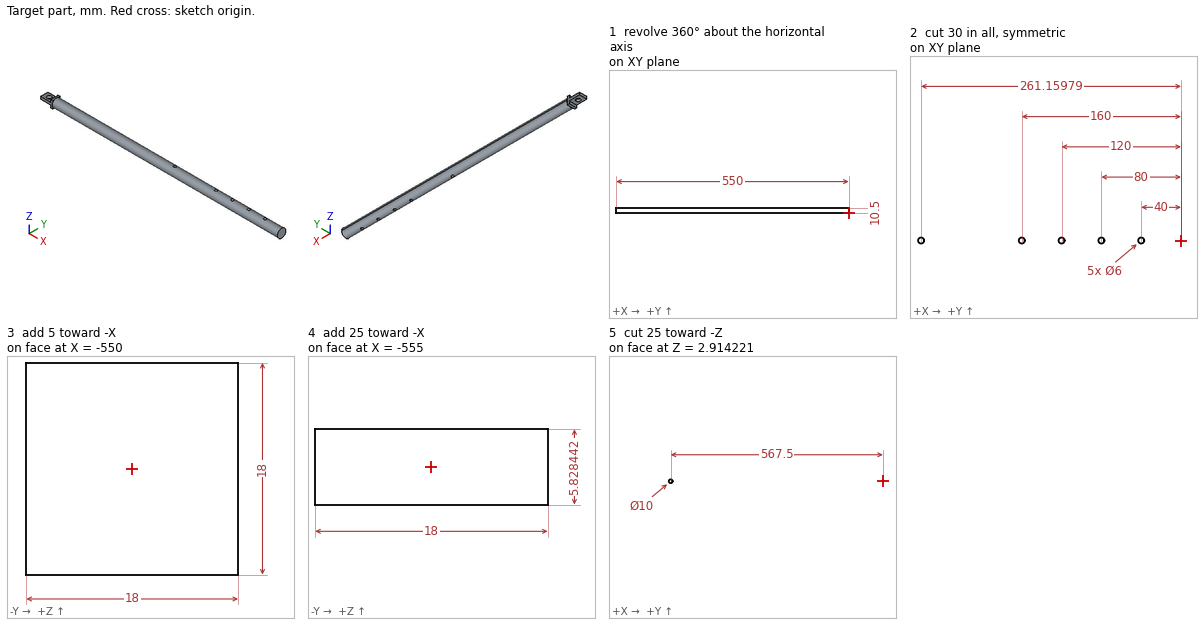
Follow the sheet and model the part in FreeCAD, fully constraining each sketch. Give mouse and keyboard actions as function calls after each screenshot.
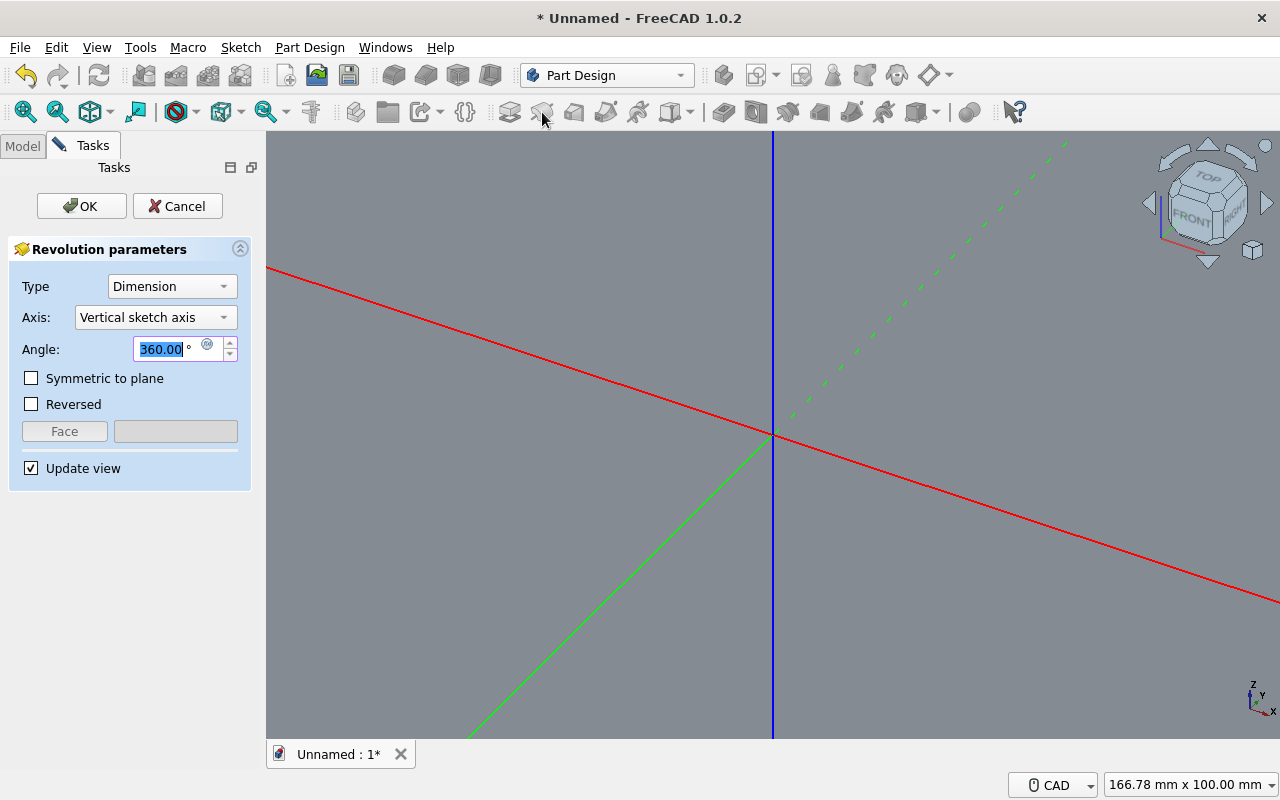
click(156, 318)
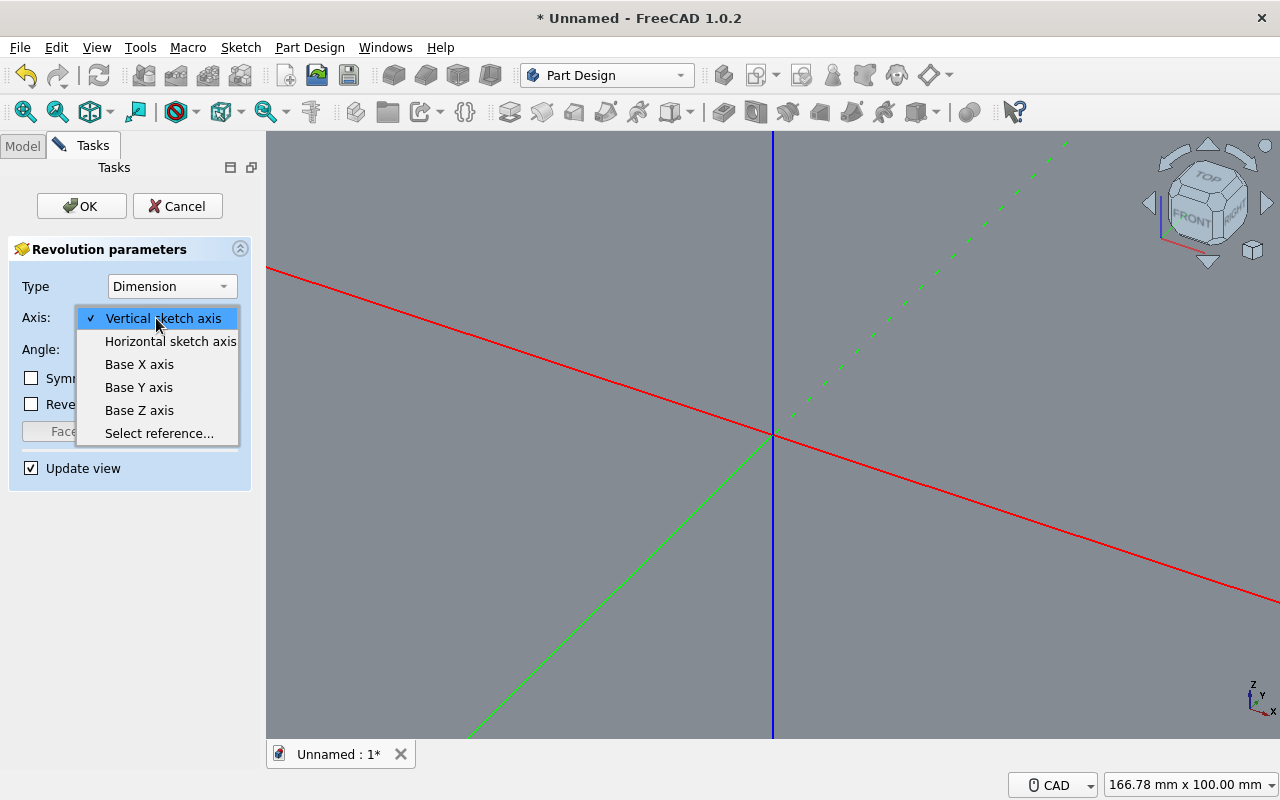
click(156, 342)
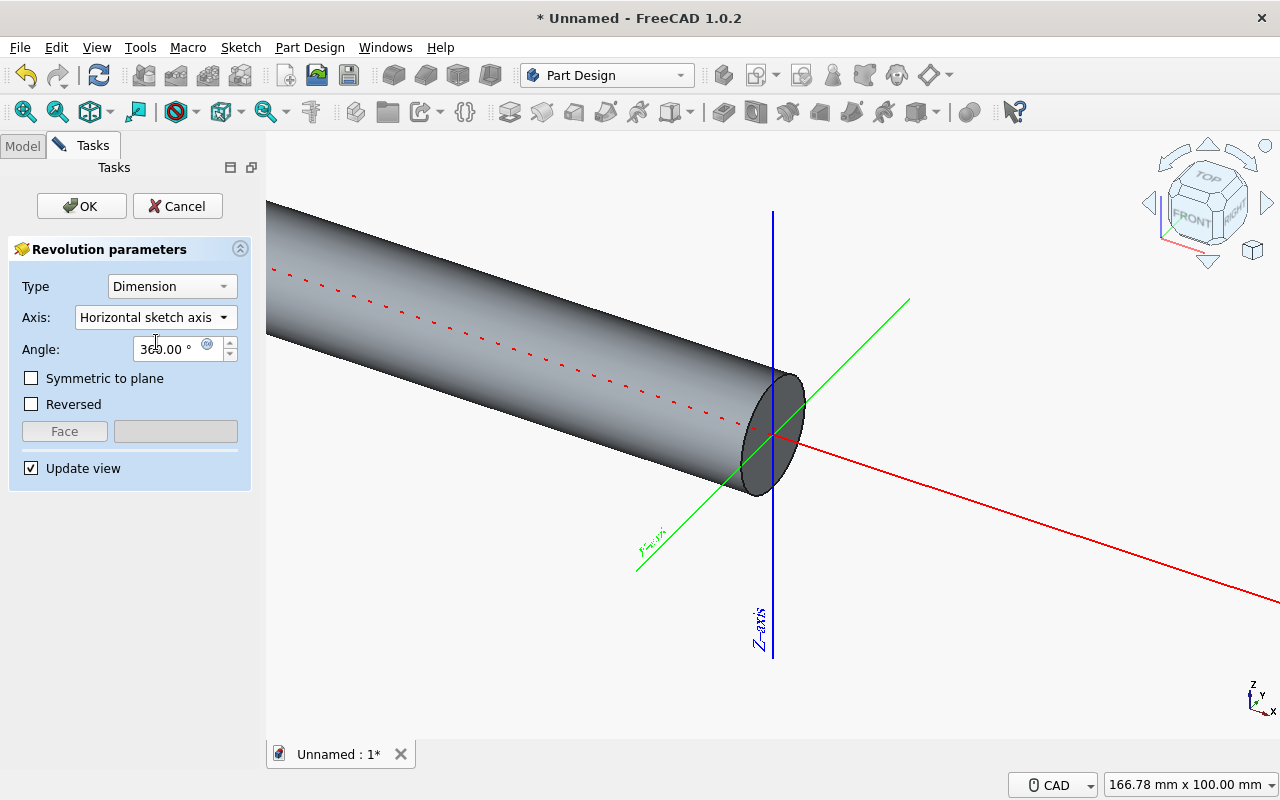
click(82, 206)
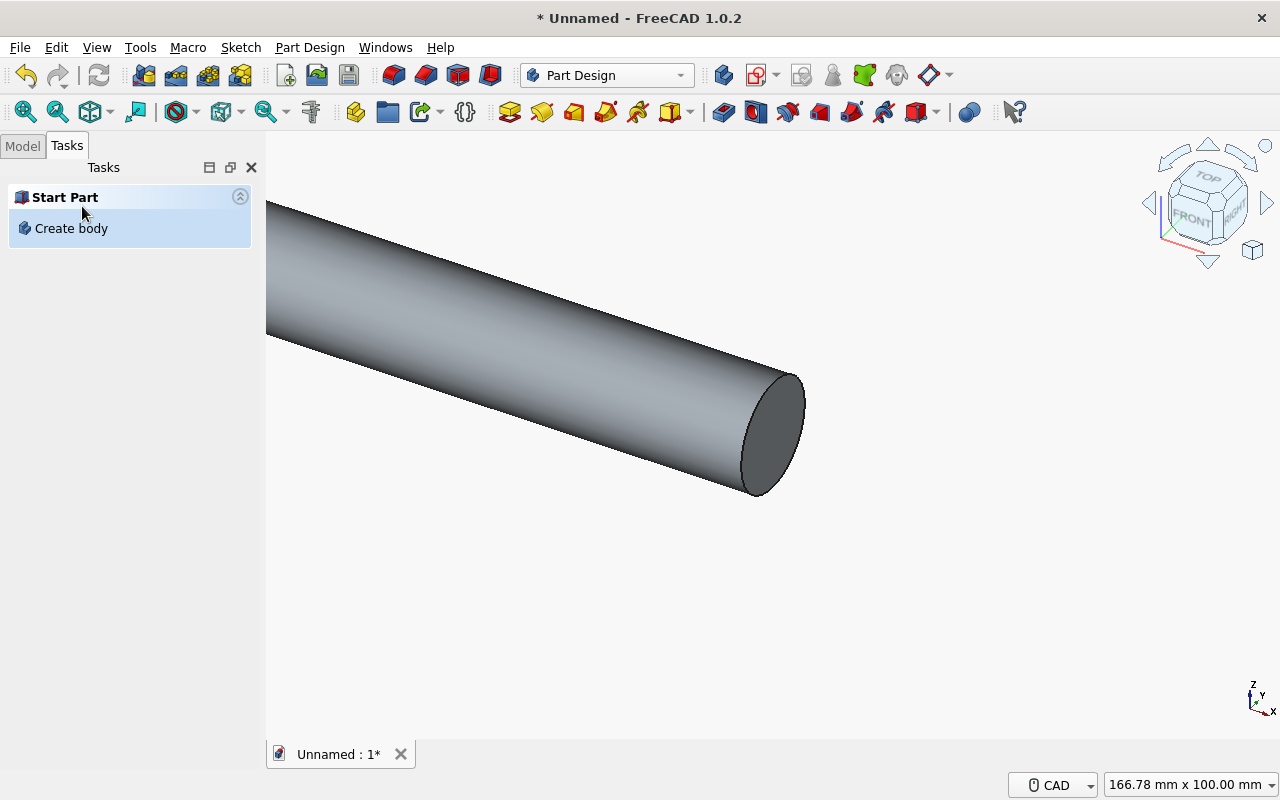
key(v)
key(f)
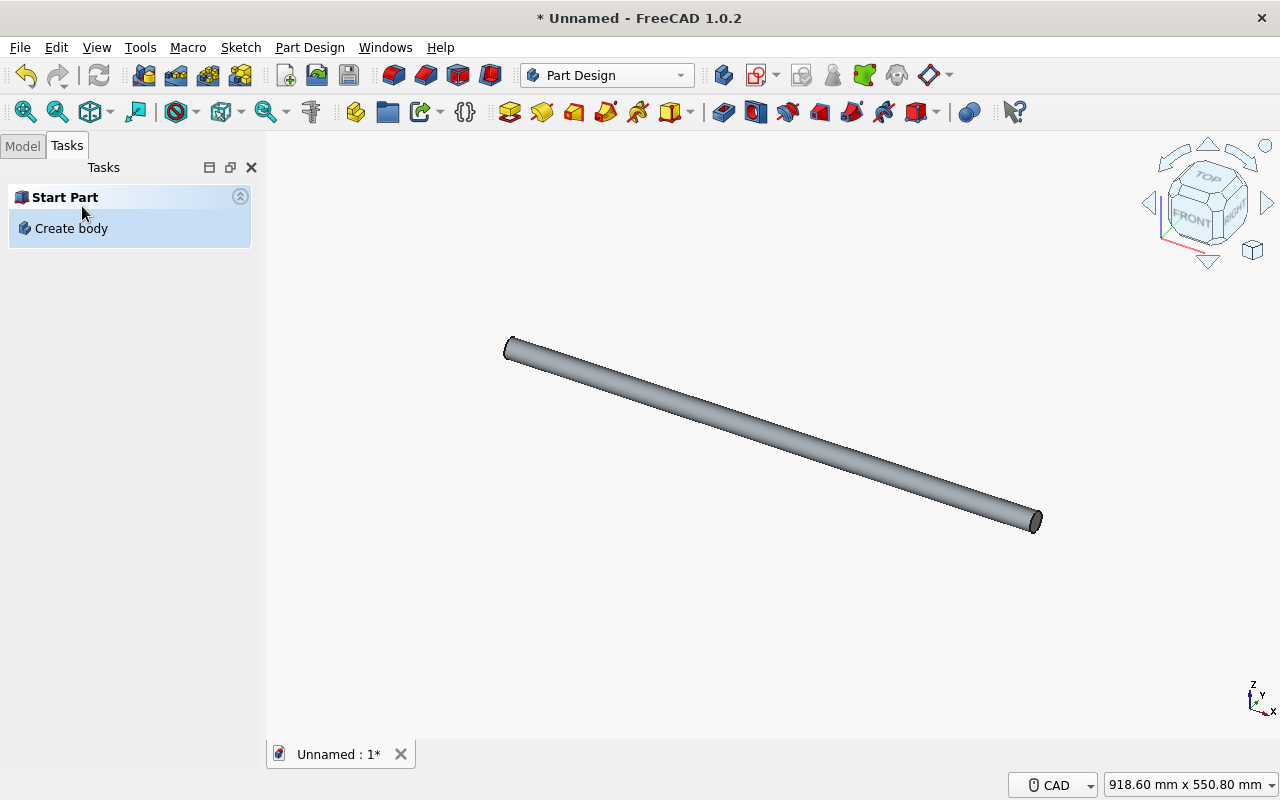
click(756, 76)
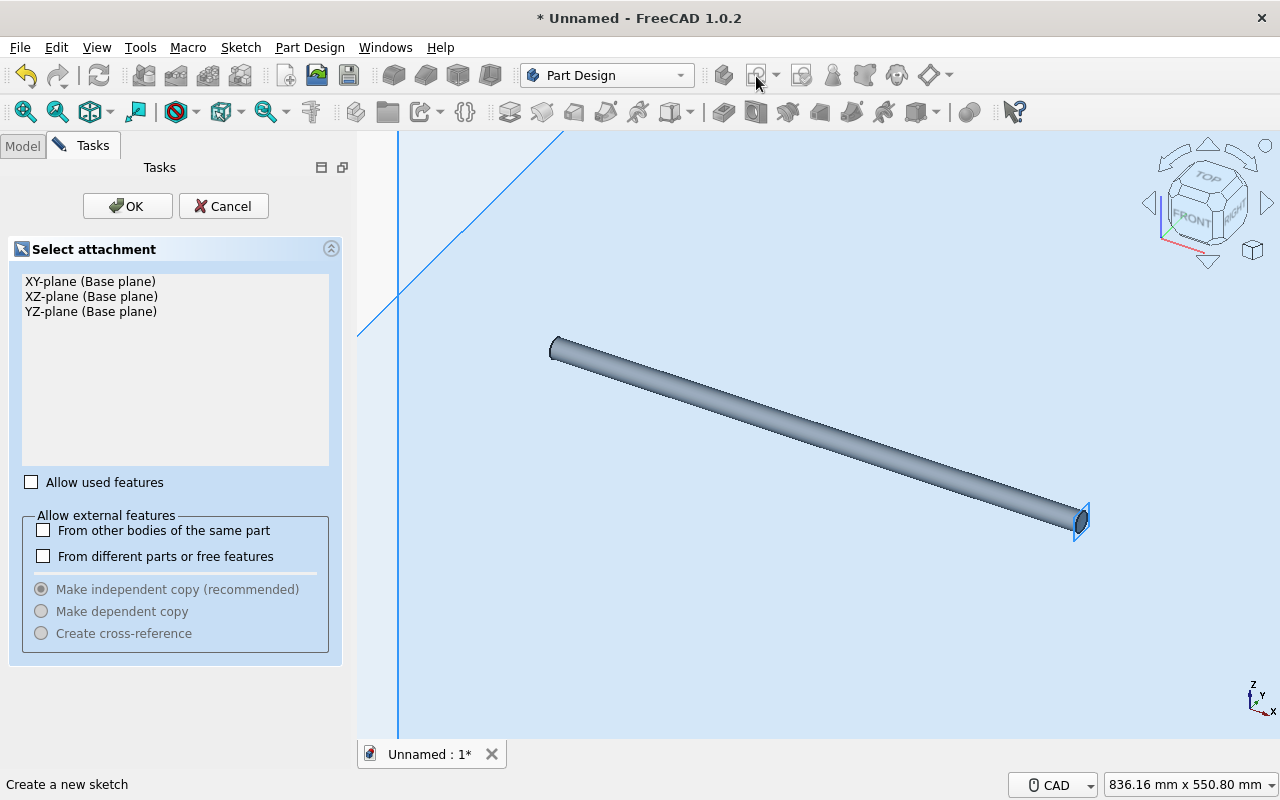
click(82, 282)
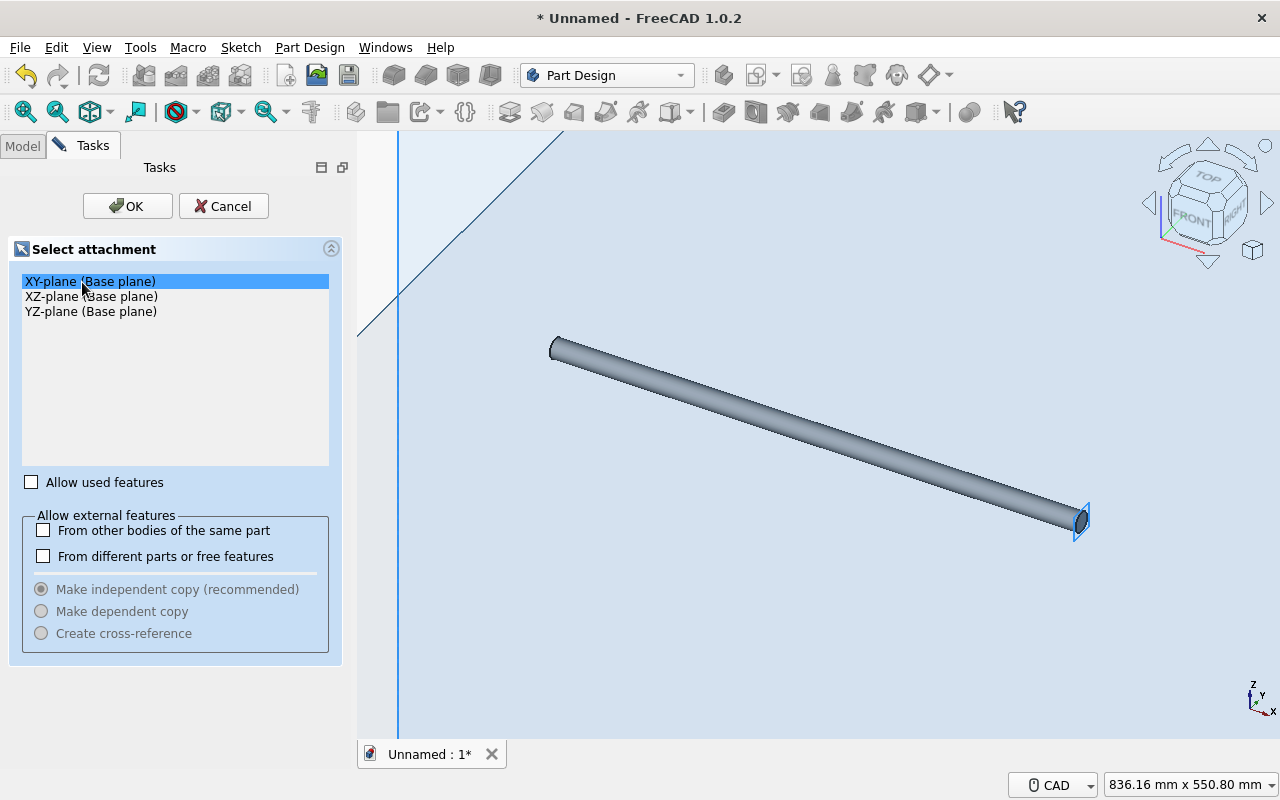
click(128, 206)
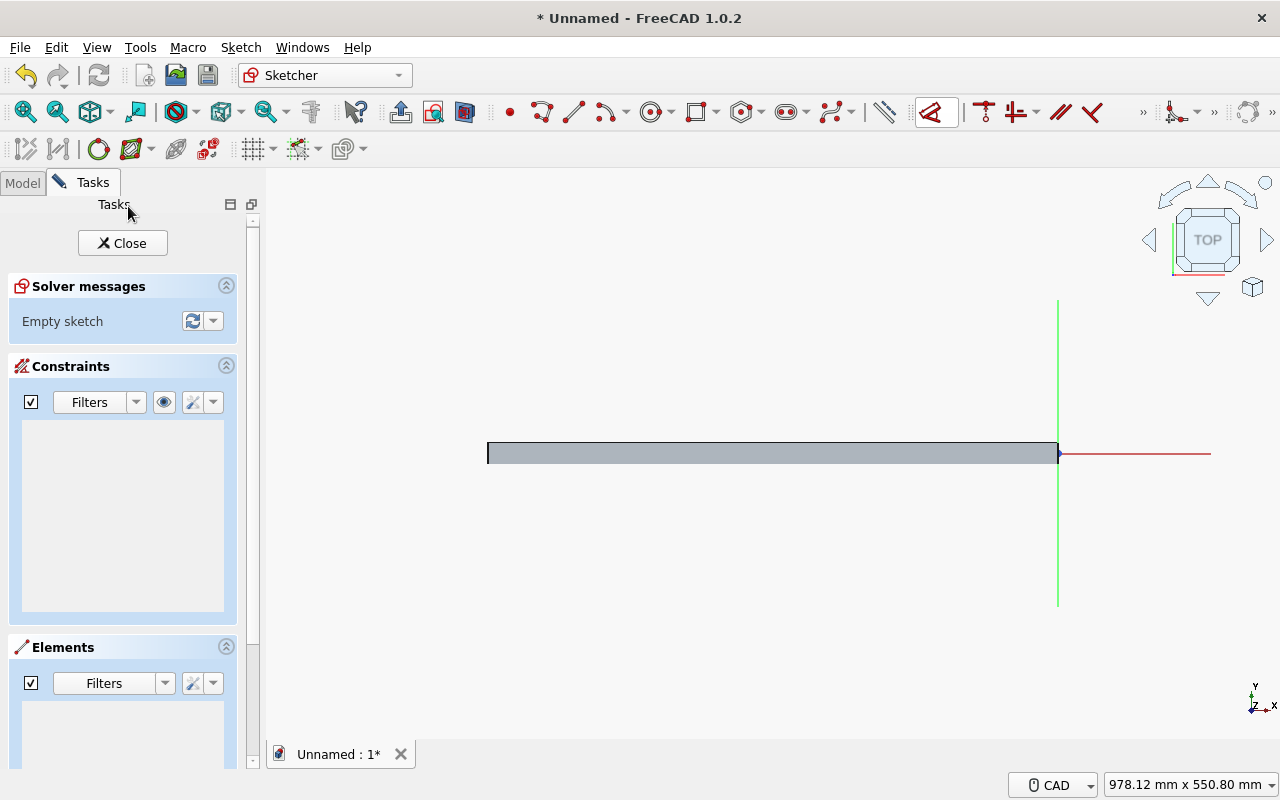
key(q)
key(s)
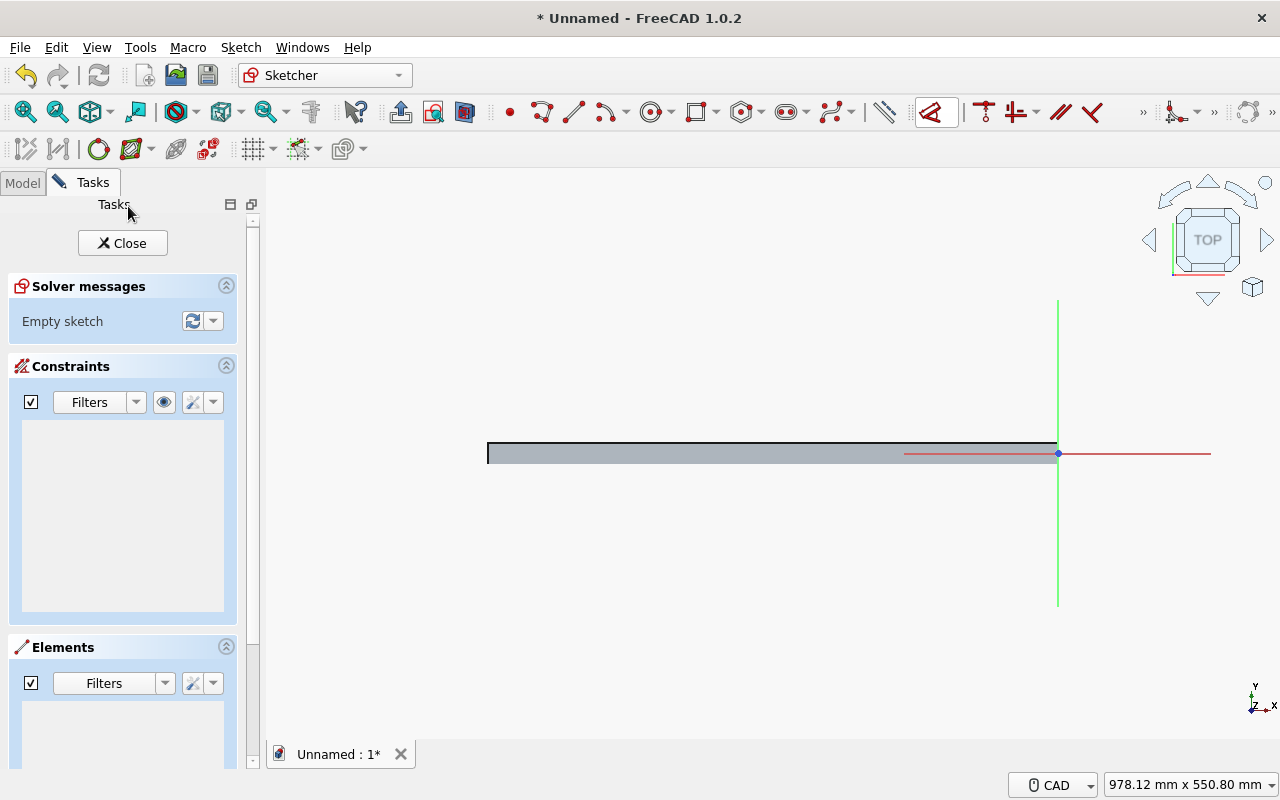
scroll(1098, 454, up, 4)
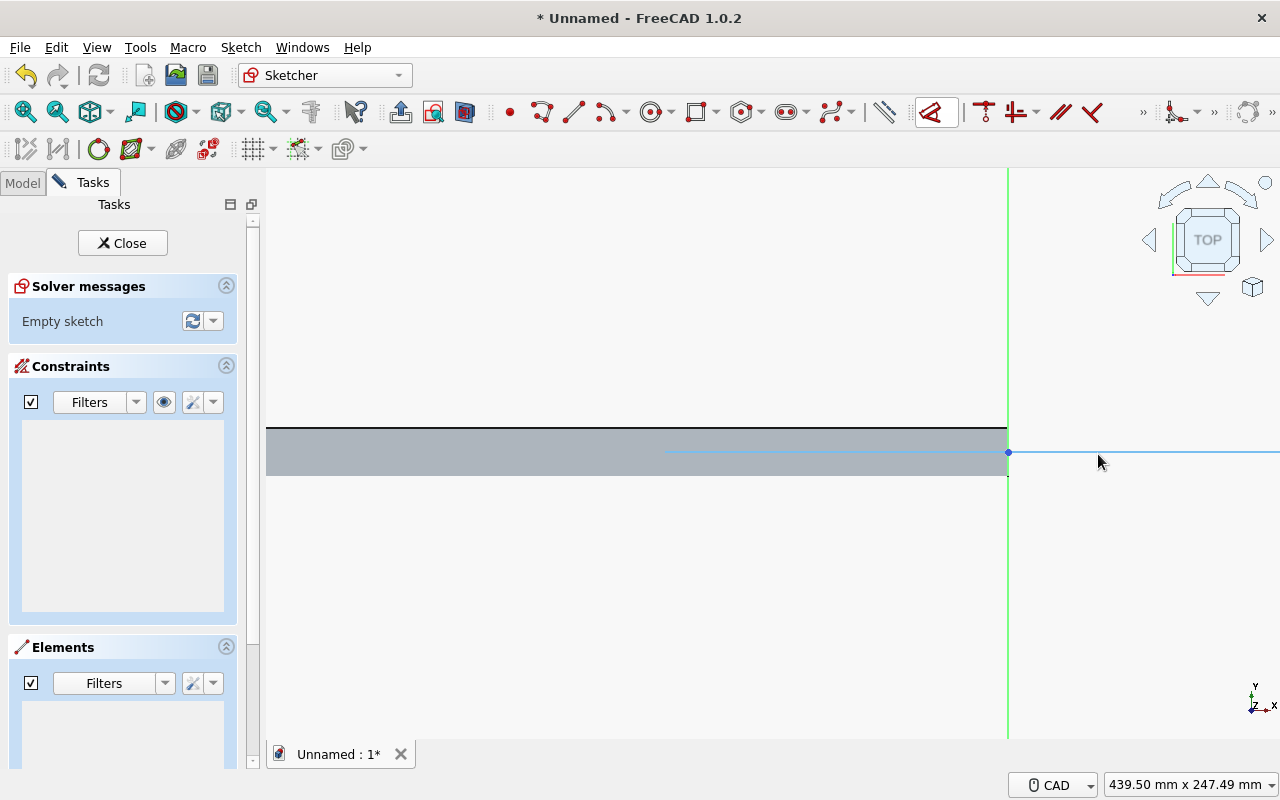
key(g)
key(c)